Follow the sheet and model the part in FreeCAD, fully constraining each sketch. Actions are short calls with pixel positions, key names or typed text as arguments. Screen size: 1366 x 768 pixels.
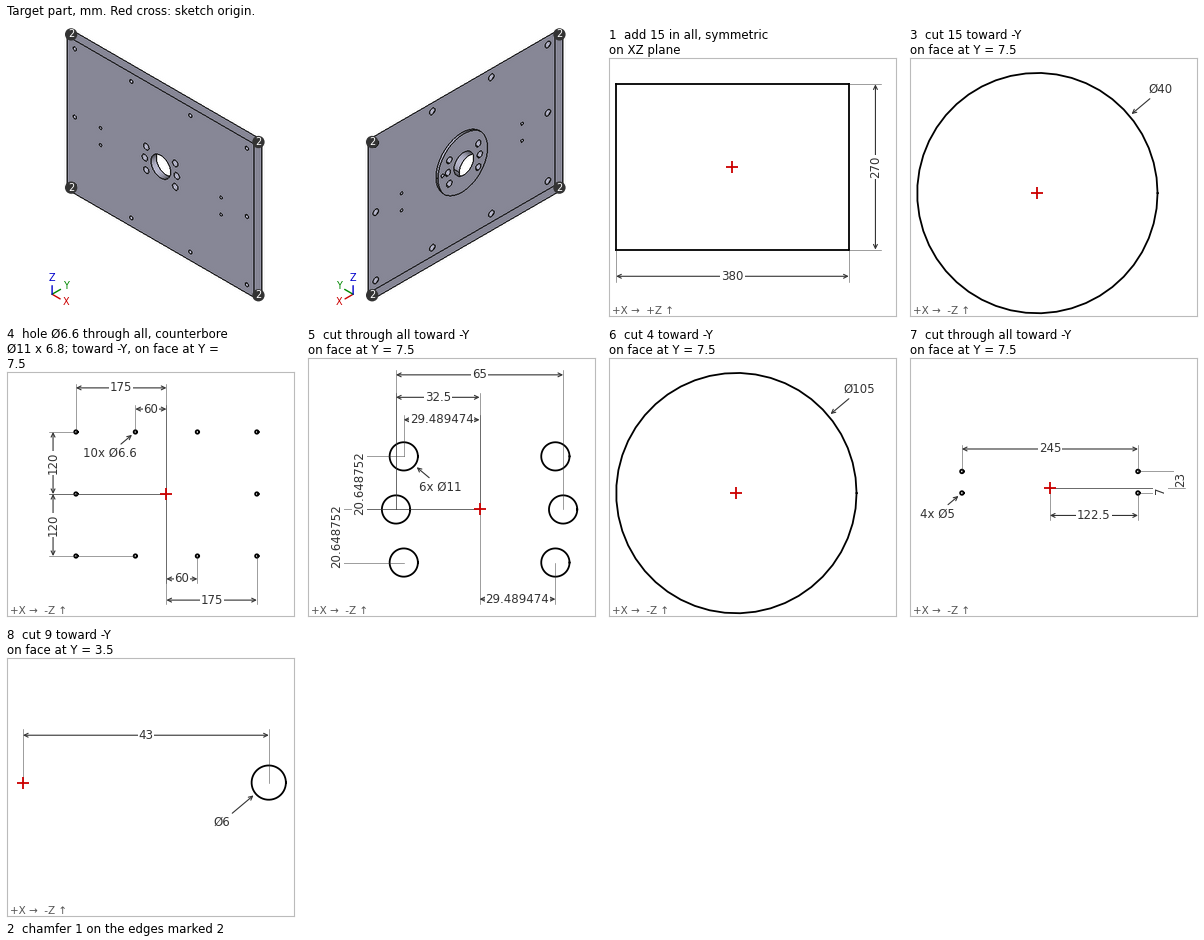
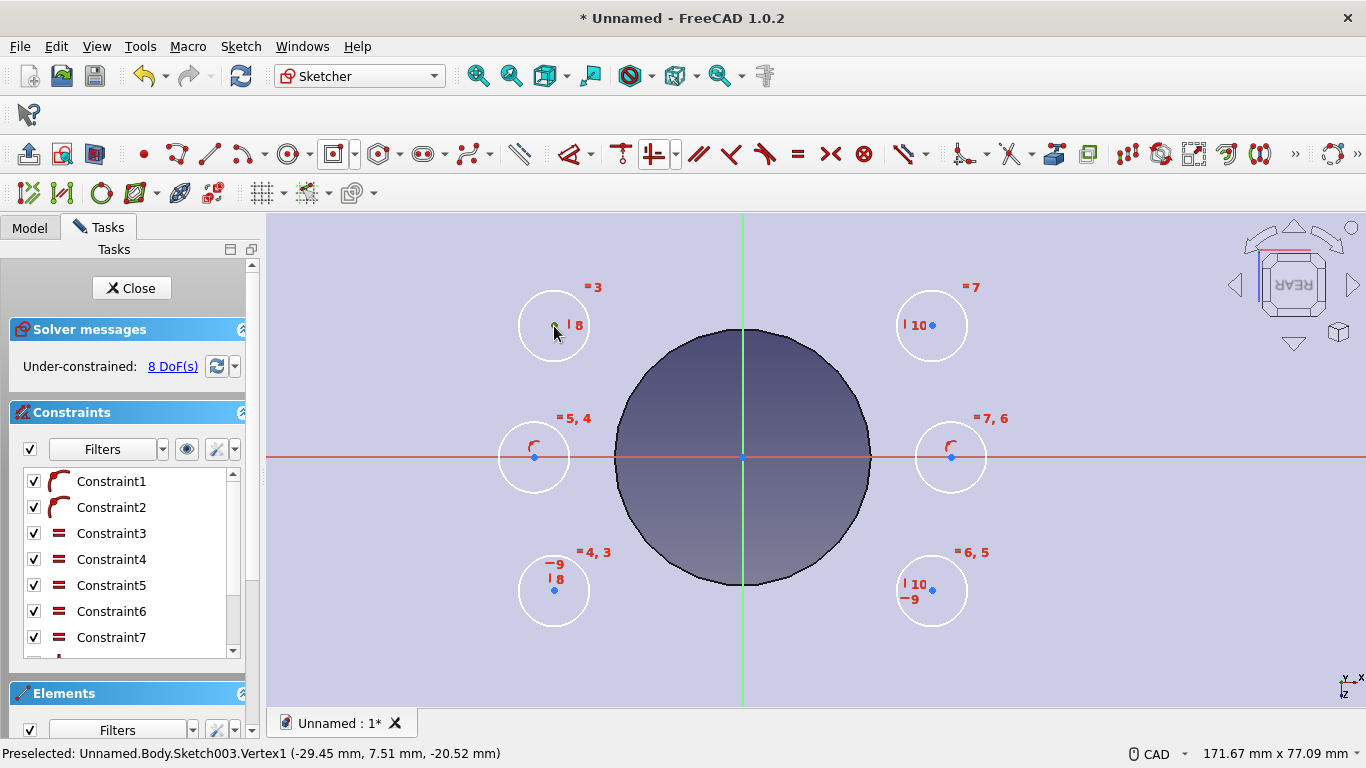
click(932, 326)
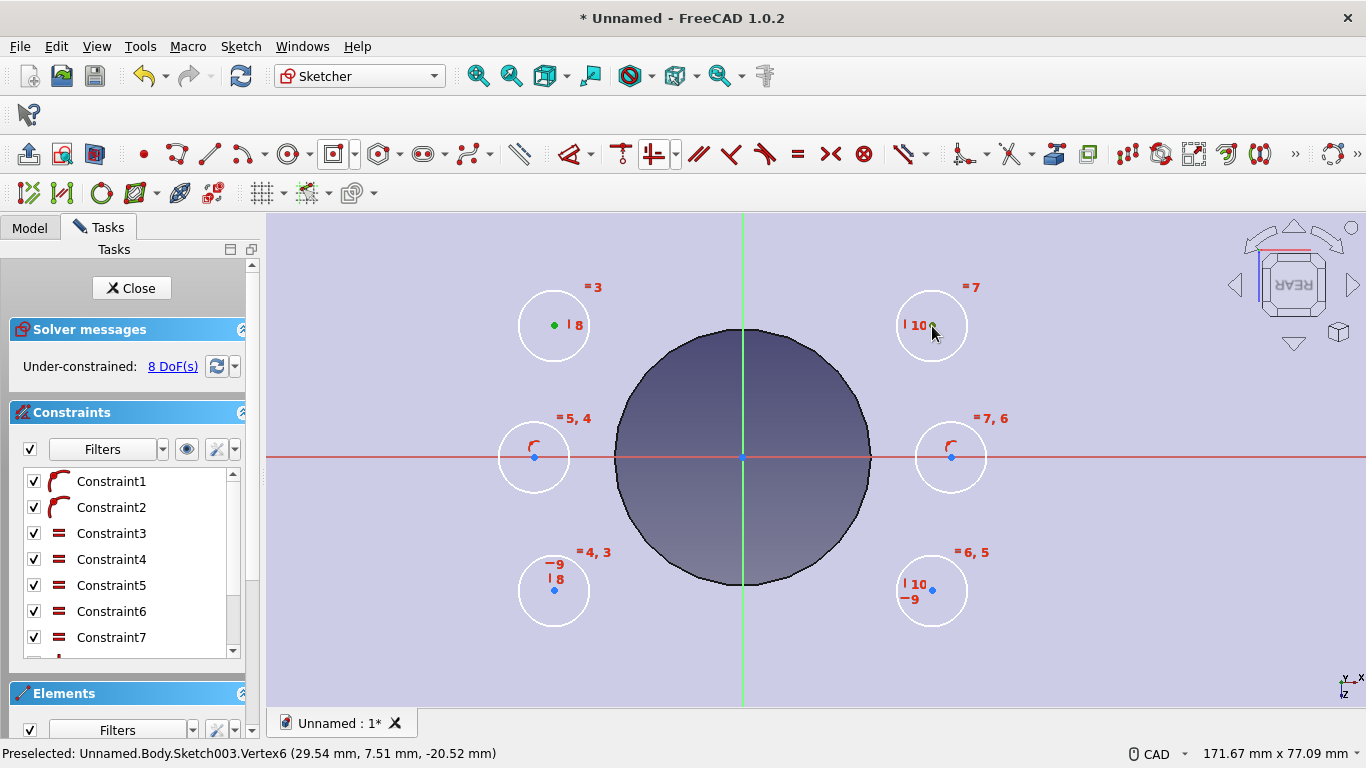
click(676, 154)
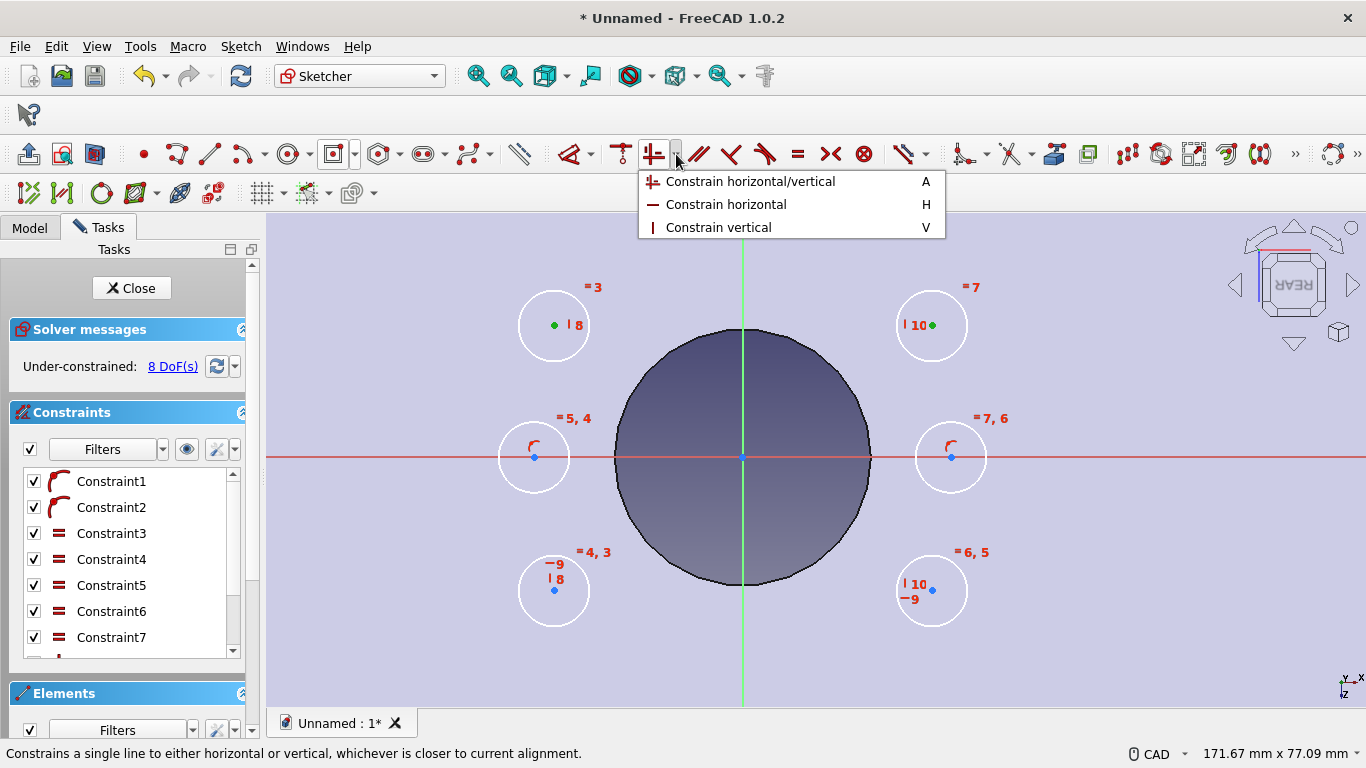
click(792, 204)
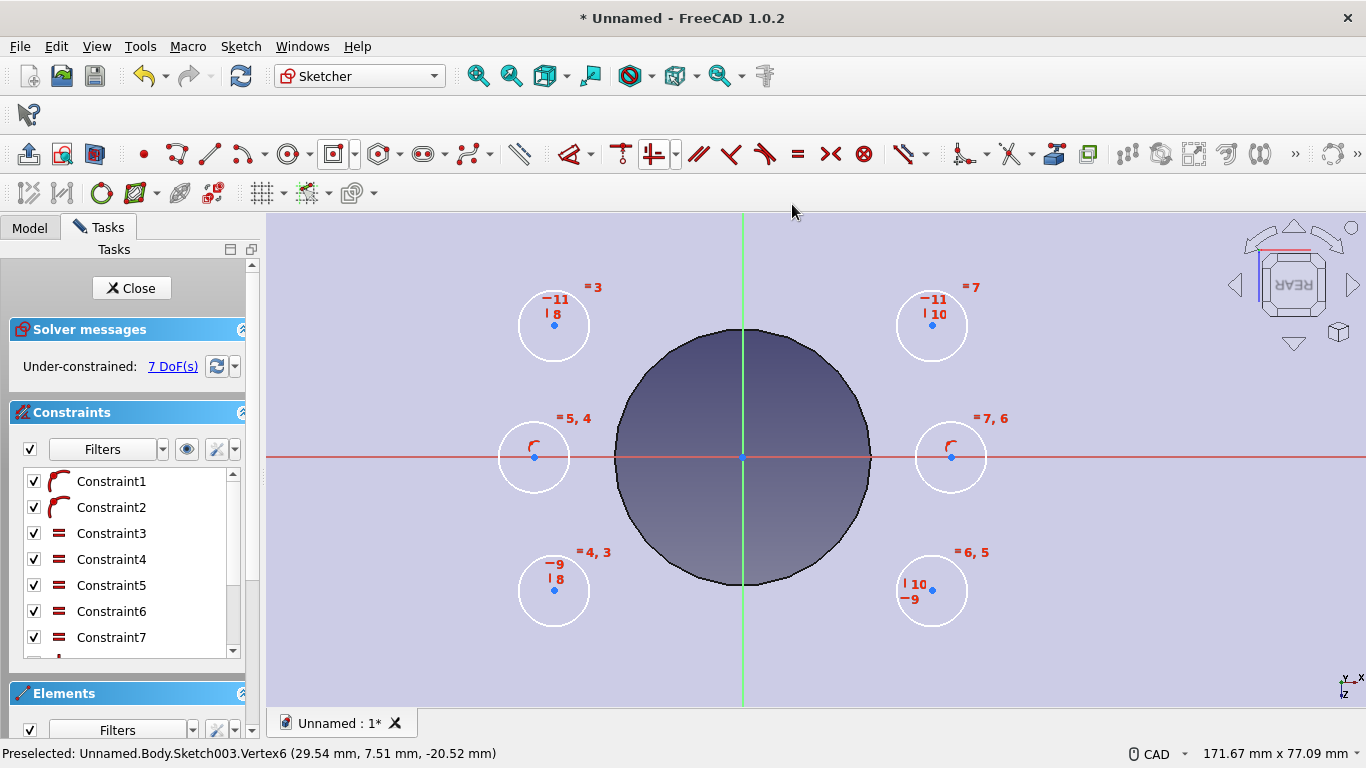
click(568, 154)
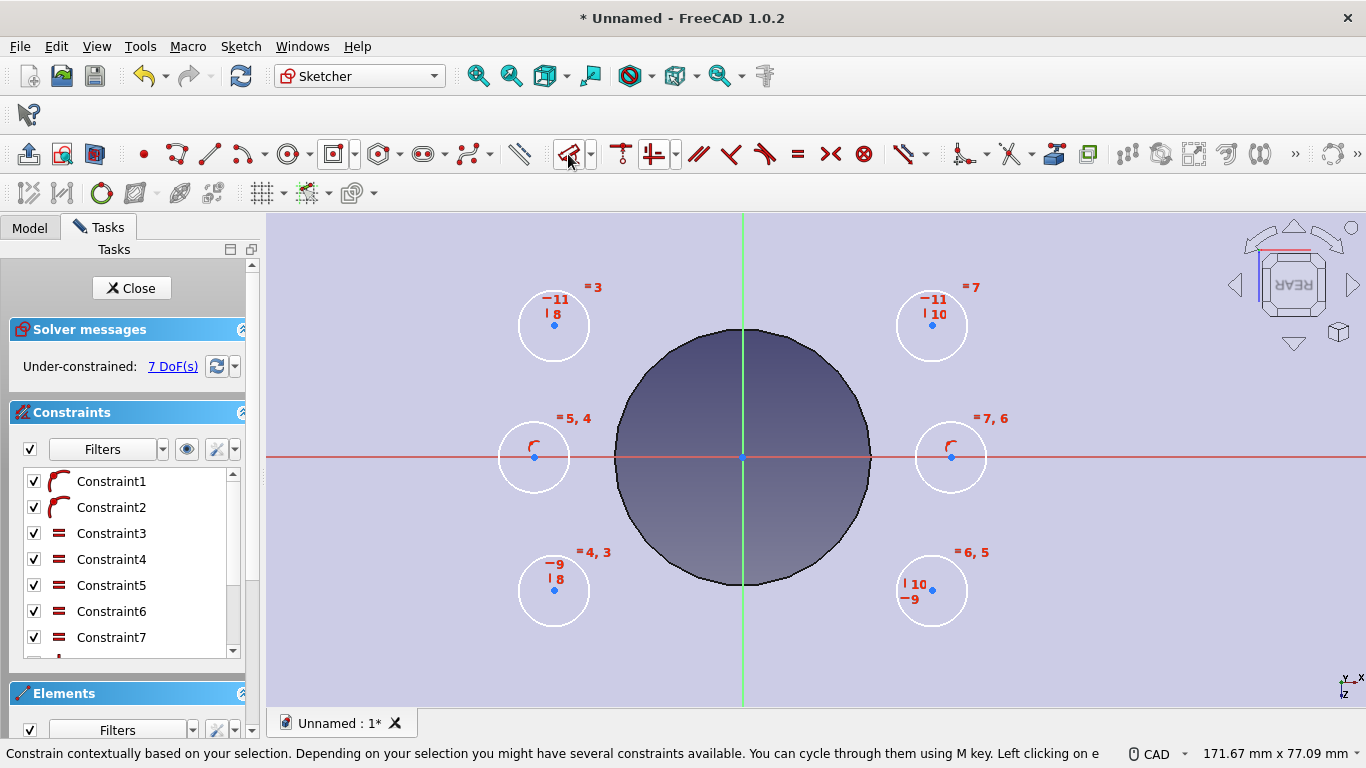
click(579, 301)
click(602, 278)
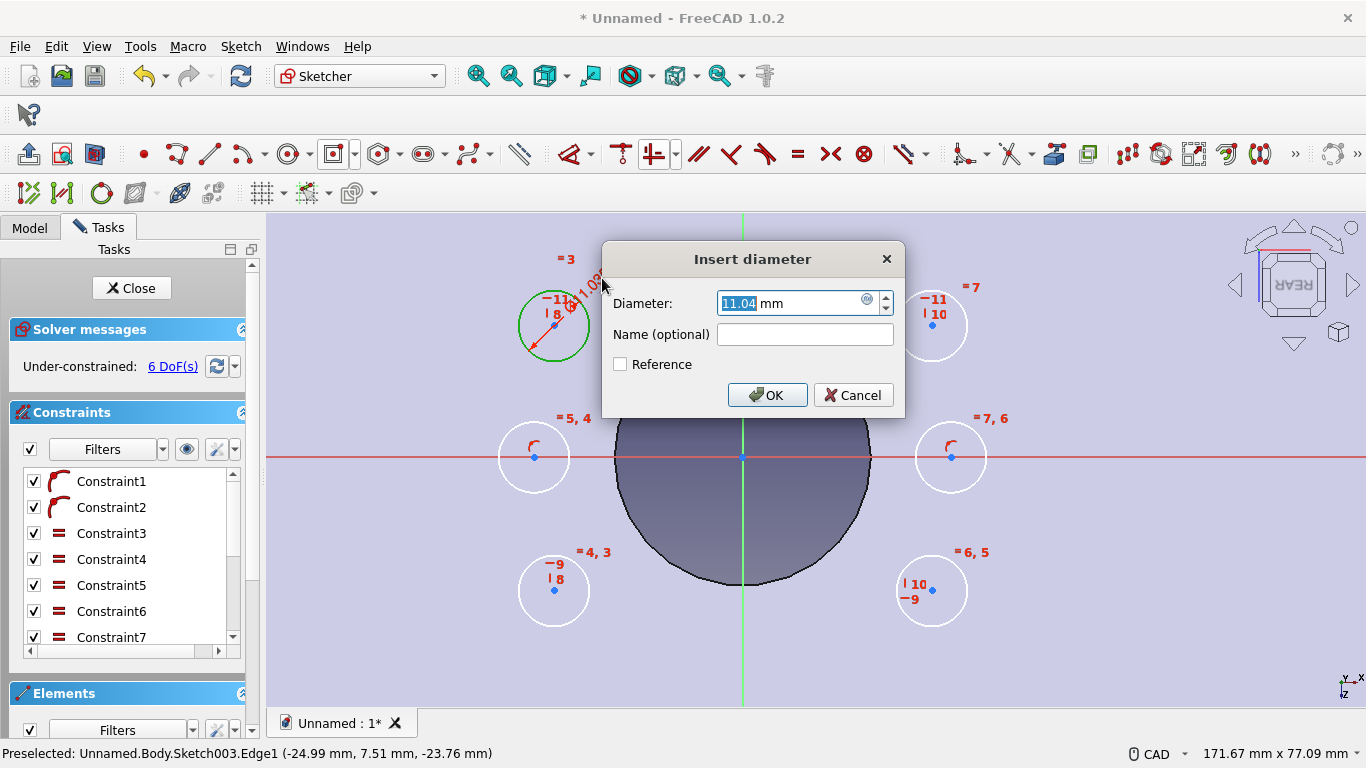
text(11)
key(Return)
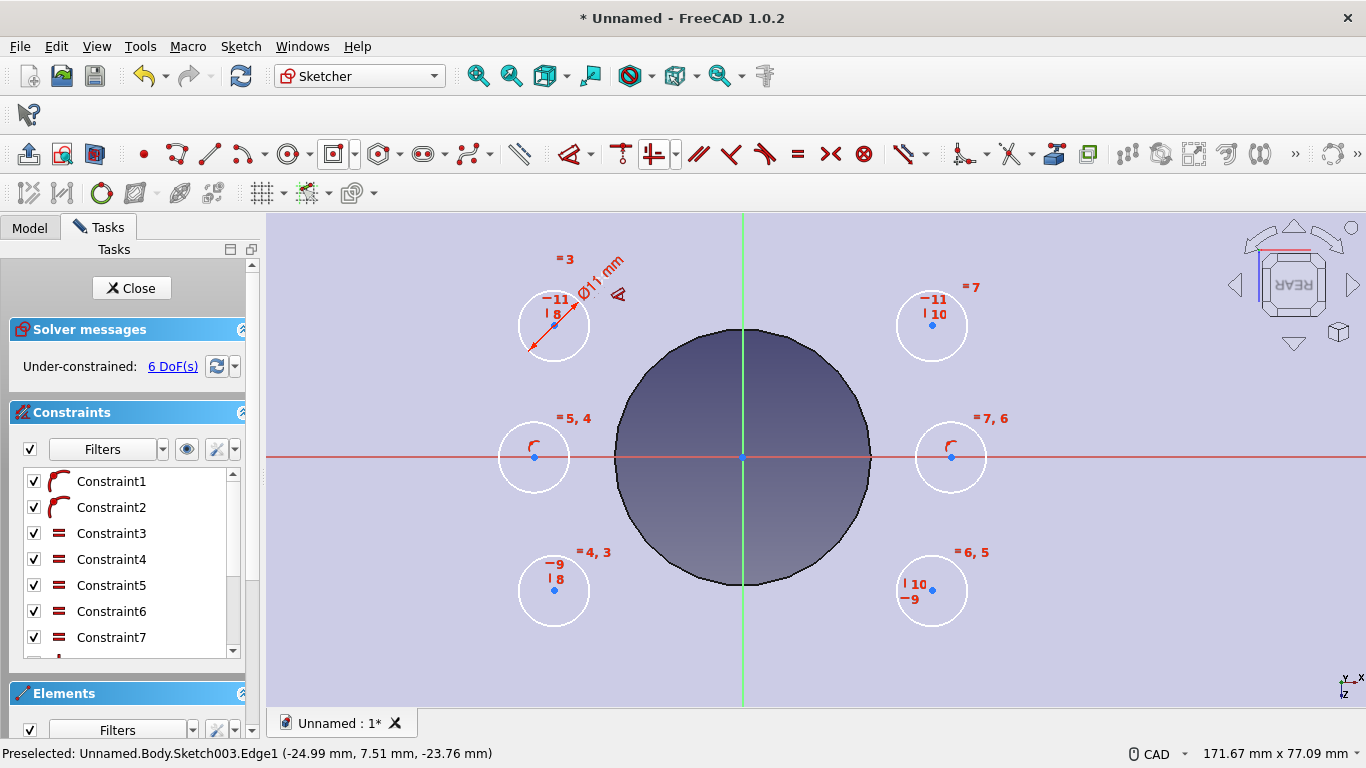
click(534, 457)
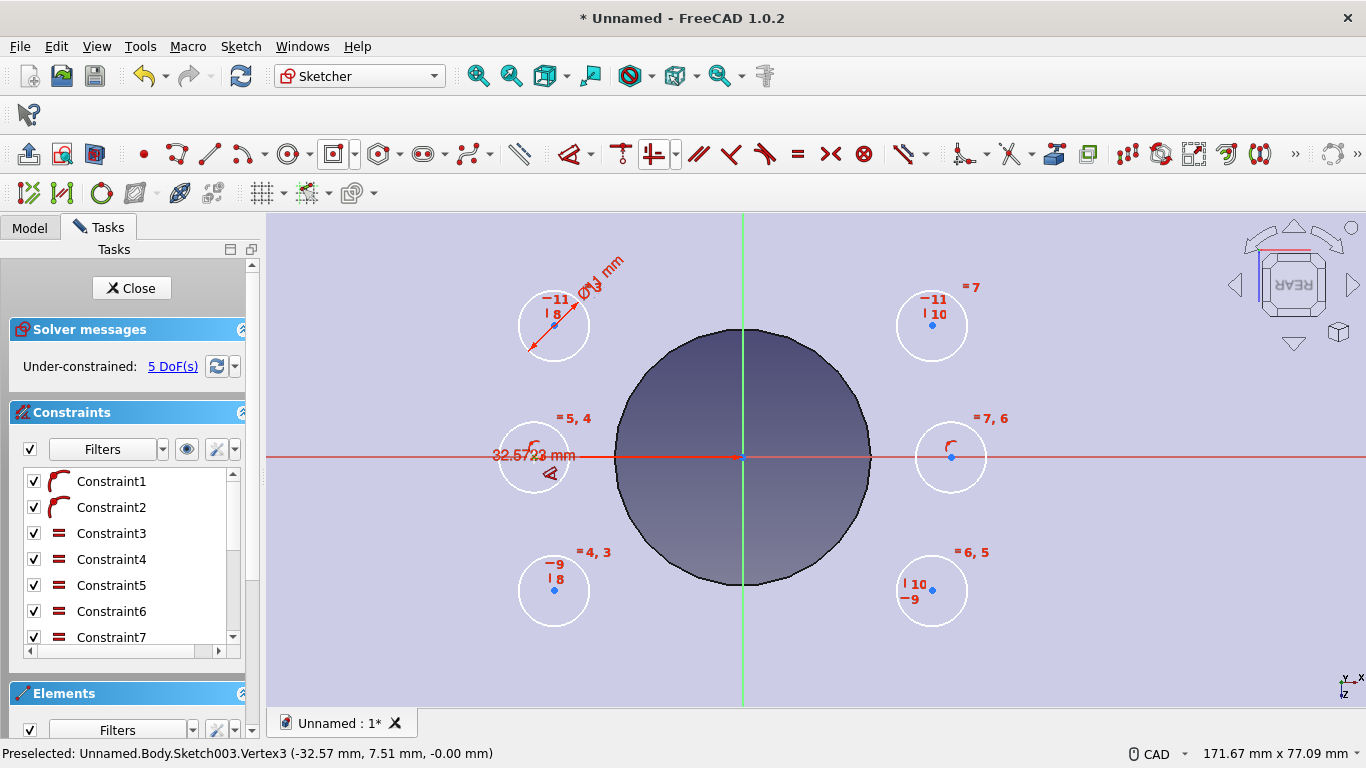
click(951, 457)
click(647, 491)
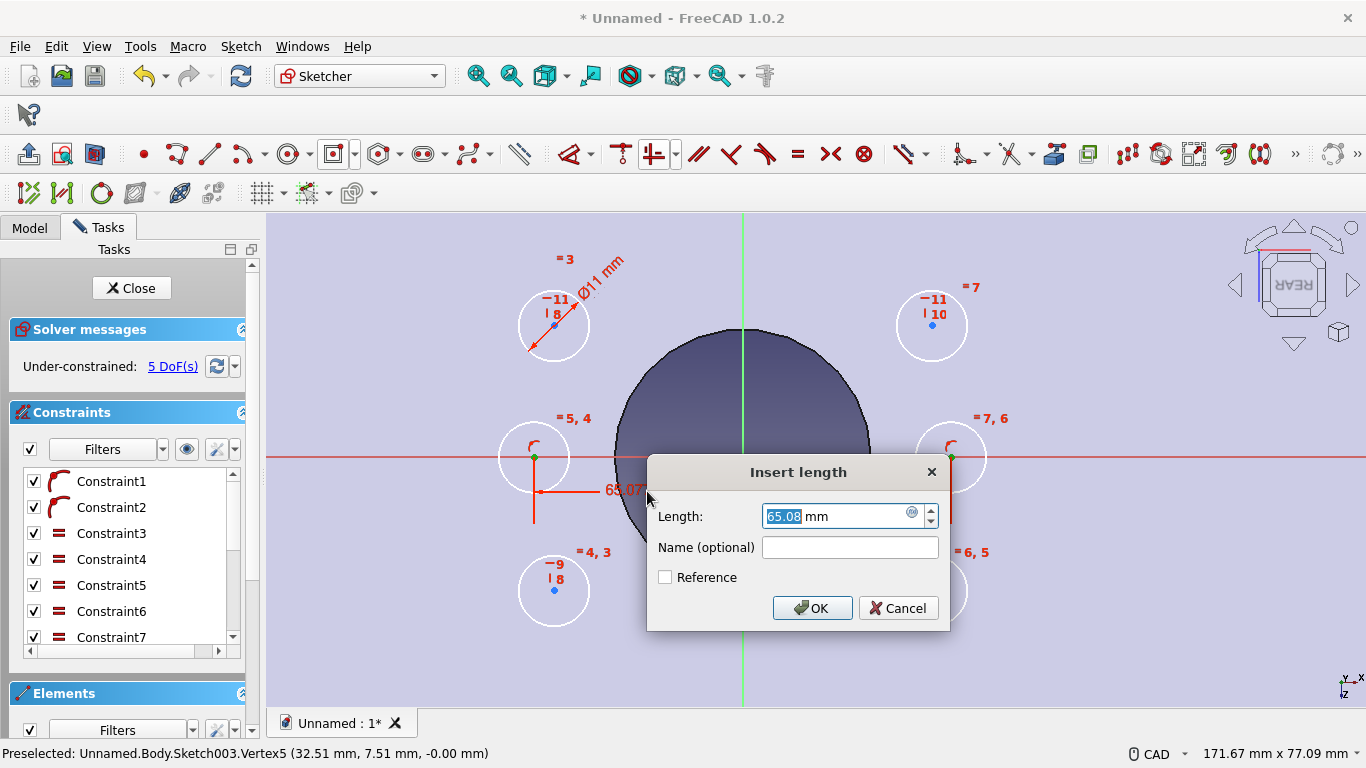
text(65)
key(Return)